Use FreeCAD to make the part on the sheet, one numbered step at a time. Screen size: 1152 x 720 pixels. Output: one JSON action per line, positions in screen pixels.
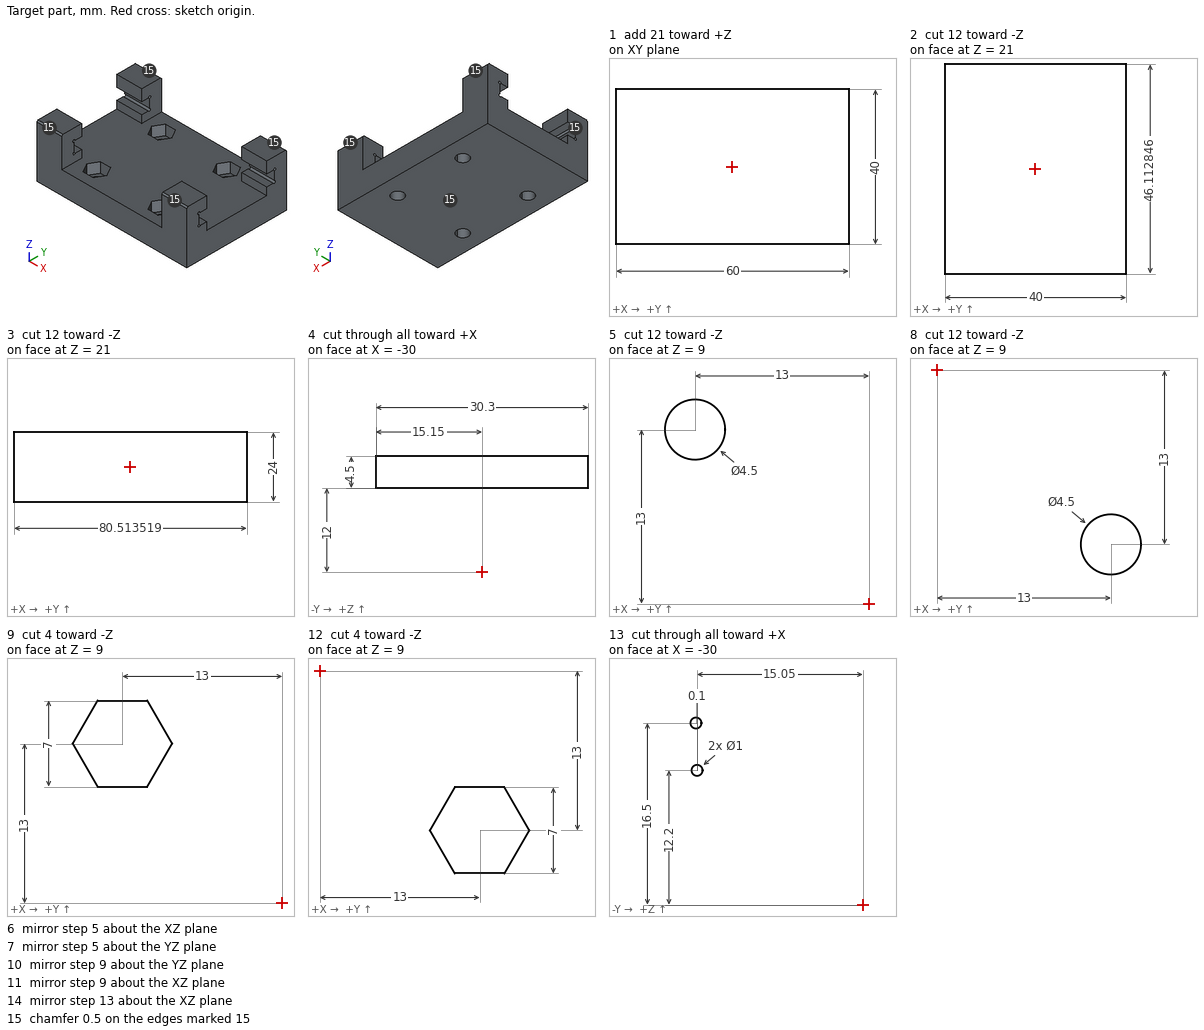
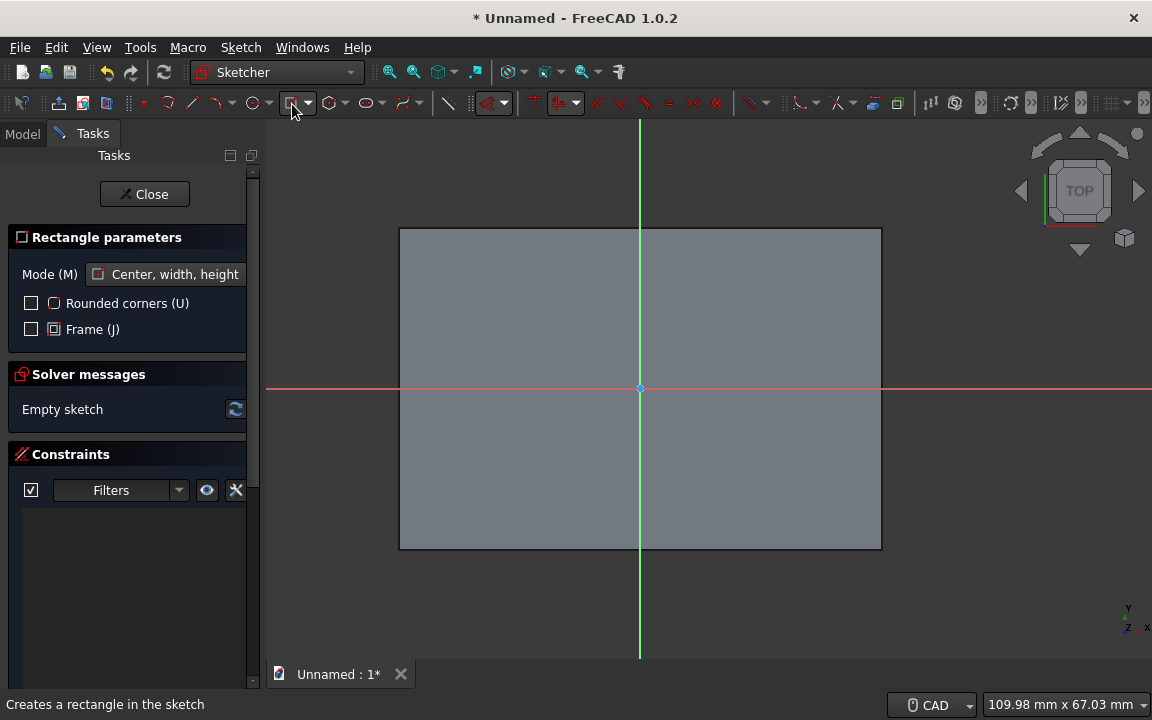
{"action": "left_click", "coordinate": [640, 389]}
{"action": "left_click", "coordinate": [801, 203]}
{"action": "key", "text": "Escape"}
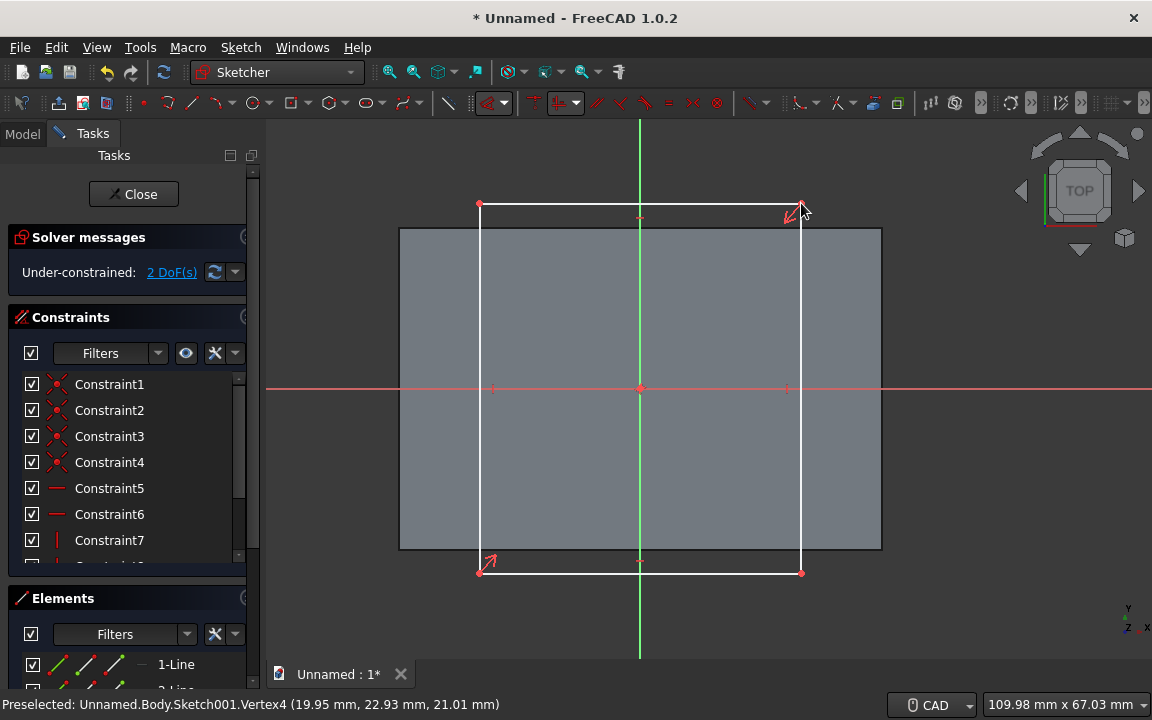
{"action": "left_click", "coordinate": [576, 574]}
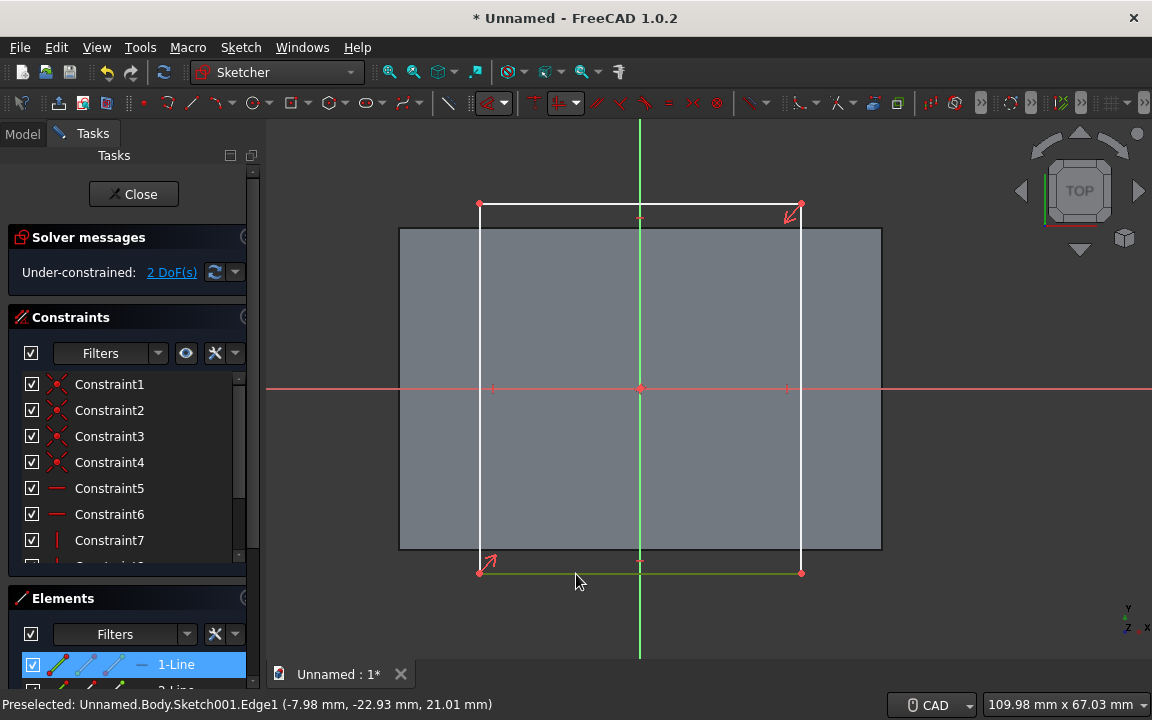
{"action": "key", "text": "l"}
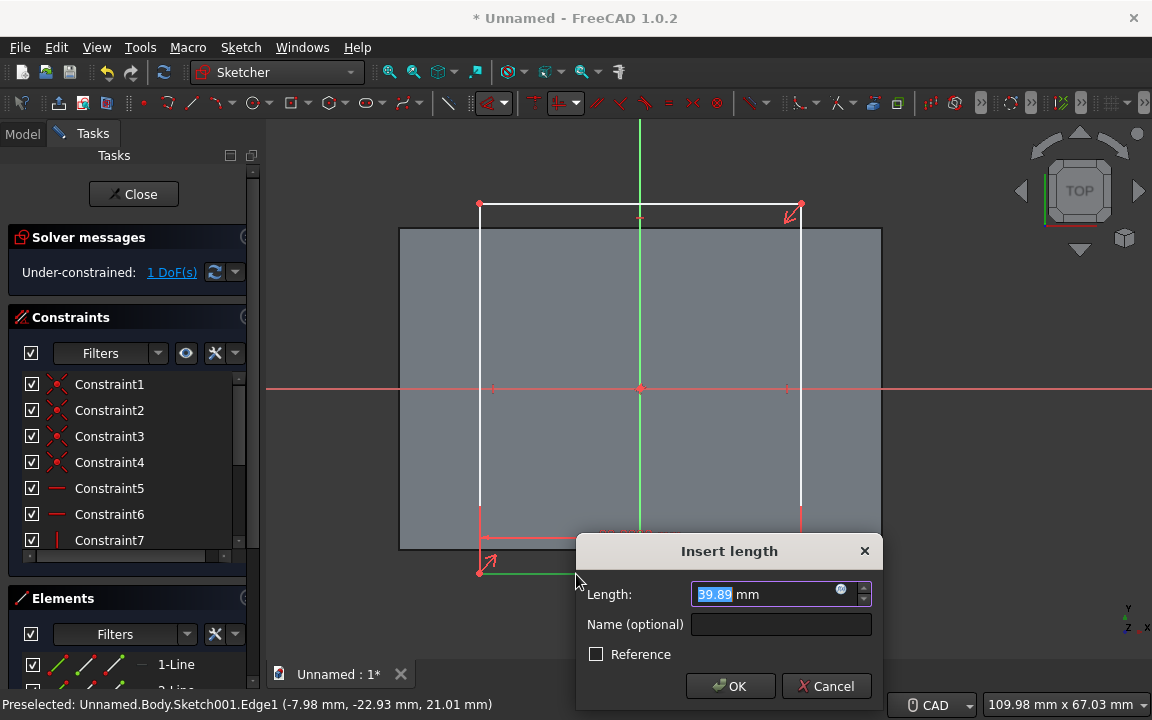
{"action": "type", "text": "40"}
{"action": "key", "text": "Return"}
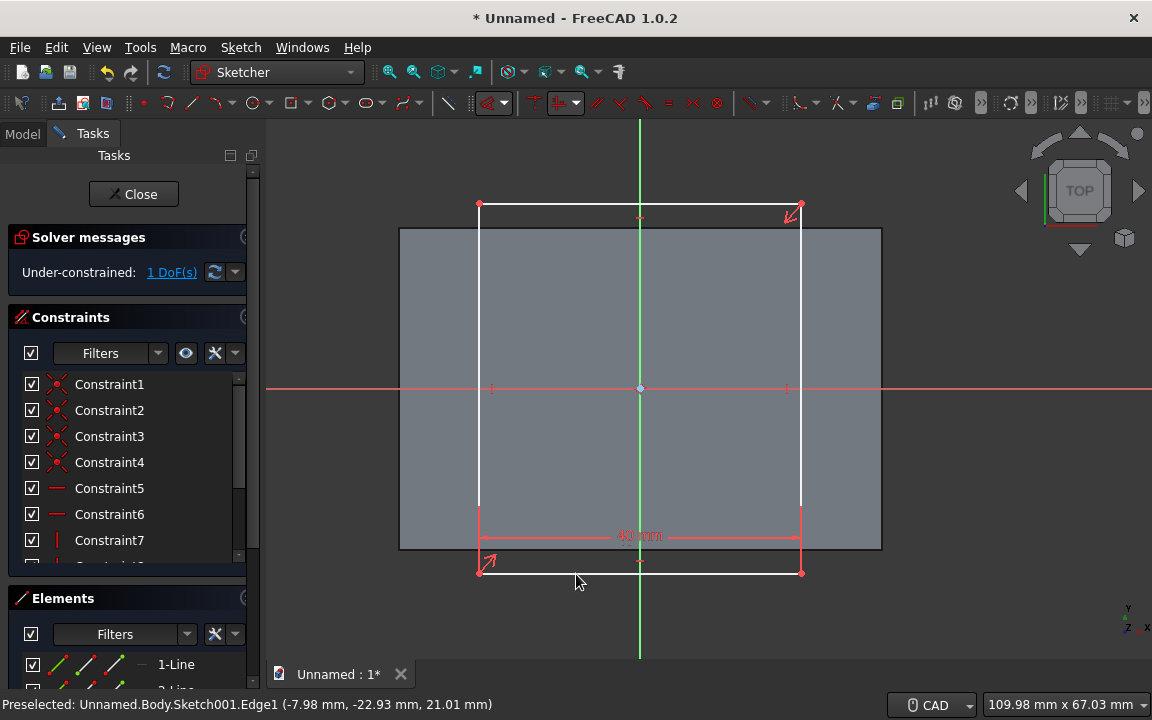
{"action": "left_click", "coordinate": [801, 463]}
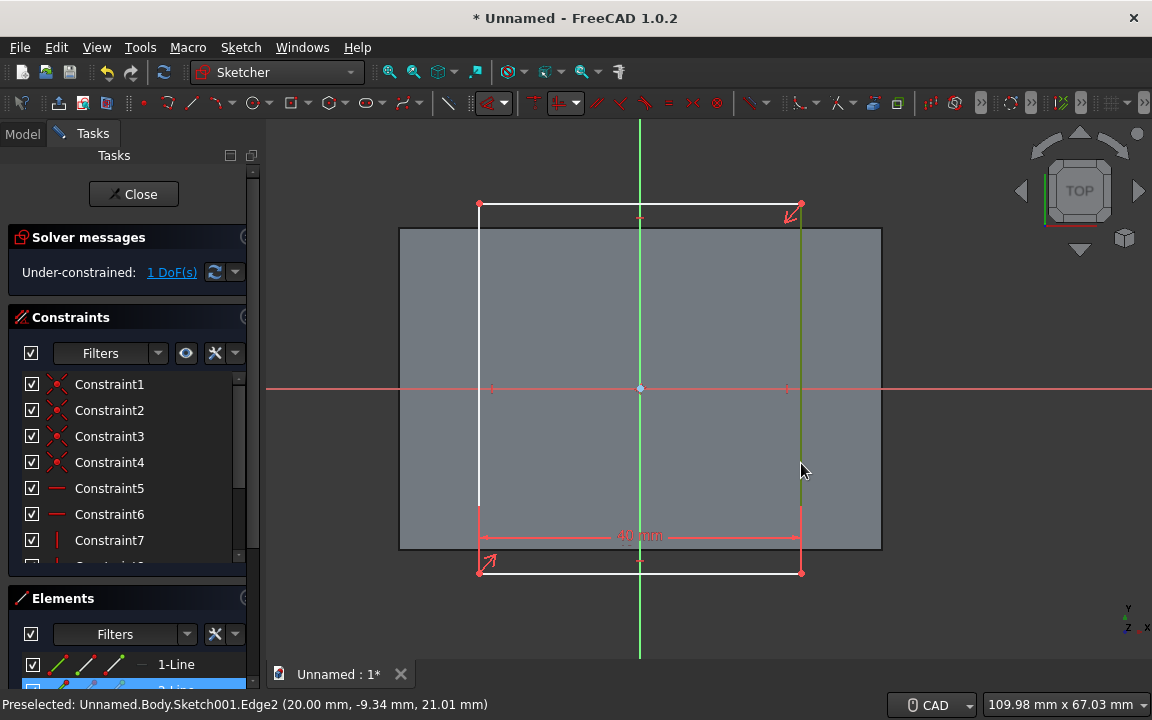
{"action": "left_click", "coordinate": [506, 104]}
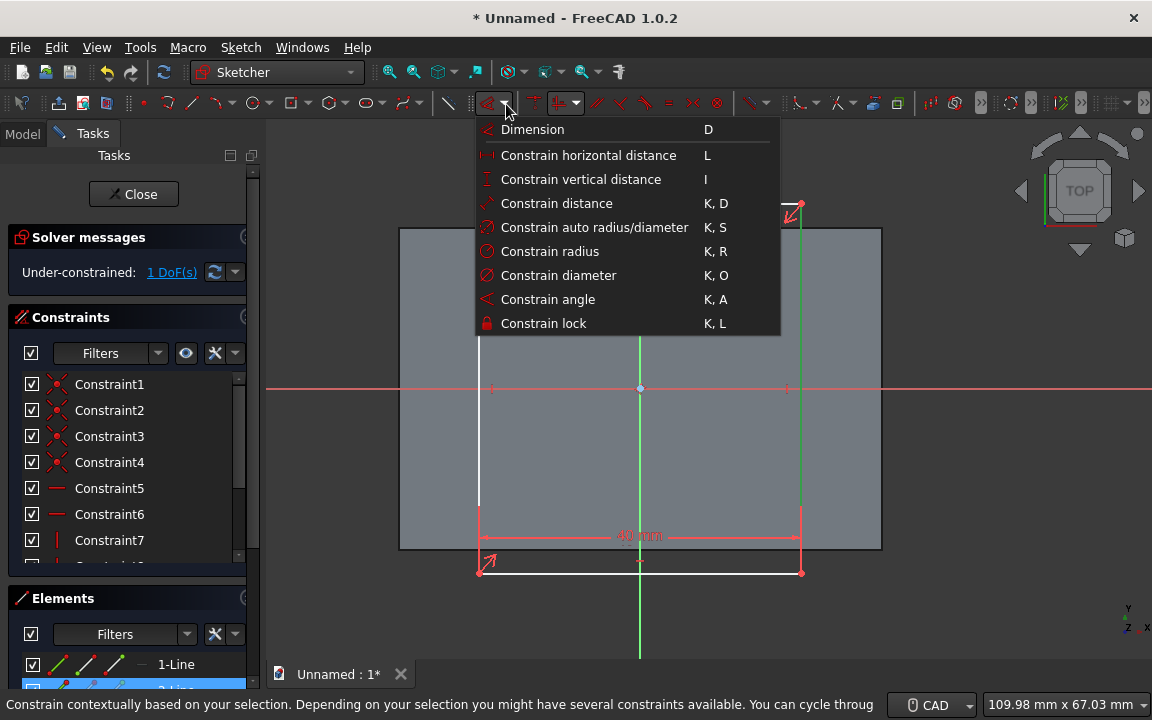
{"action": "left_click", "coordinate": [628, 179]}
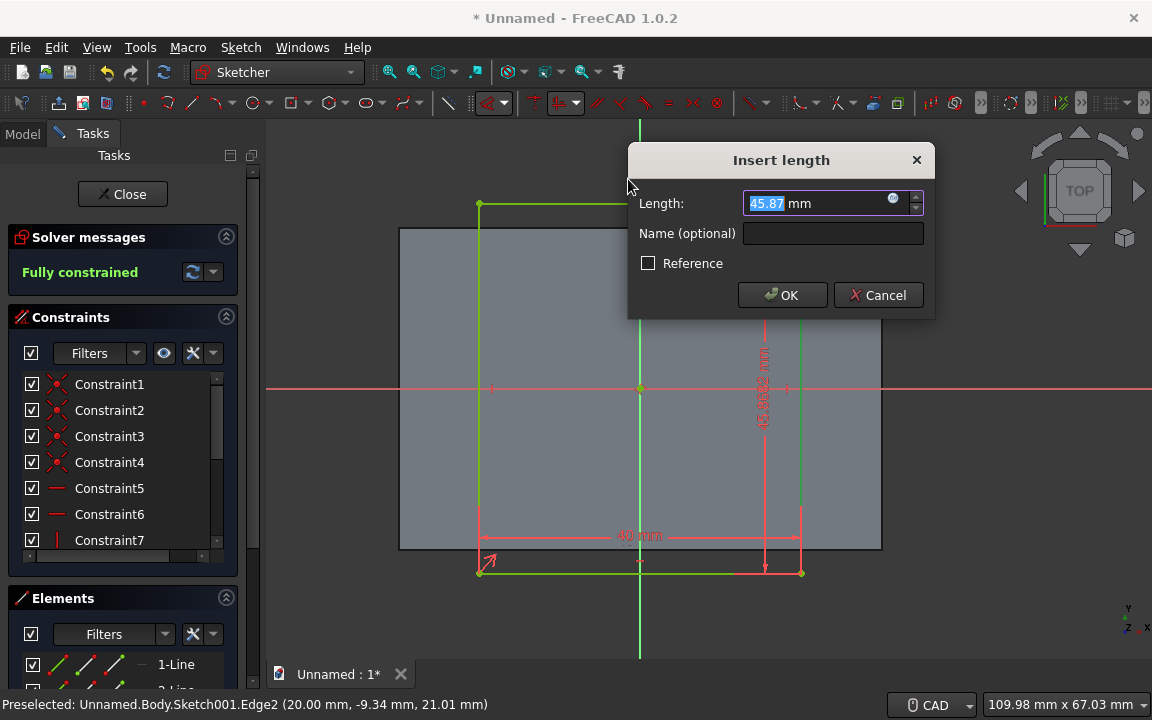
{"action": "type", "text": "46.112846"}
{"action": "key", "text": "Return"}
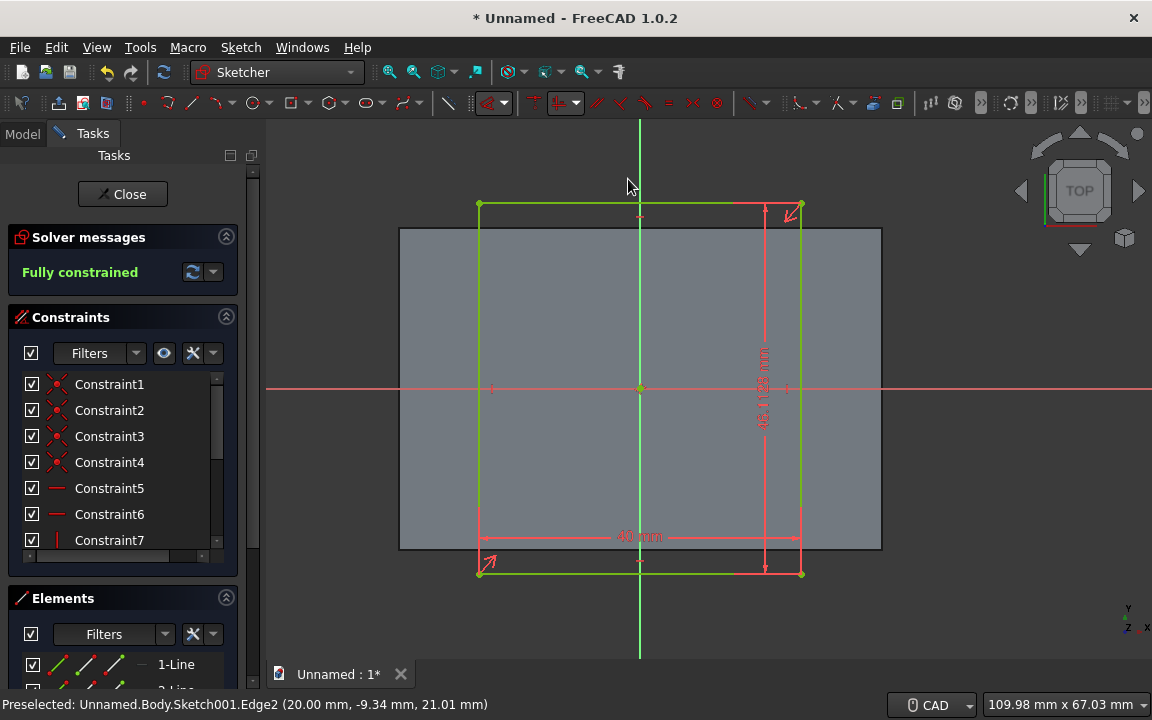
{"action": "left_click", "coordinate": [123, 194]}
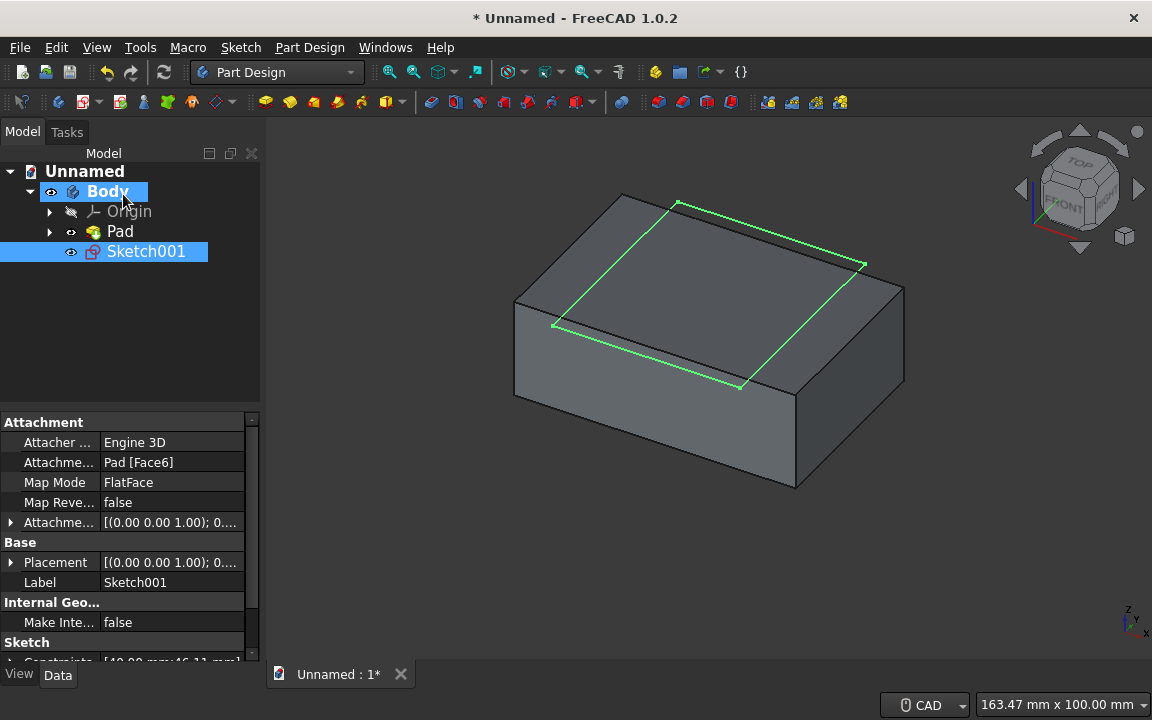
{"action": "left_click", "coordinate": [432, 102]}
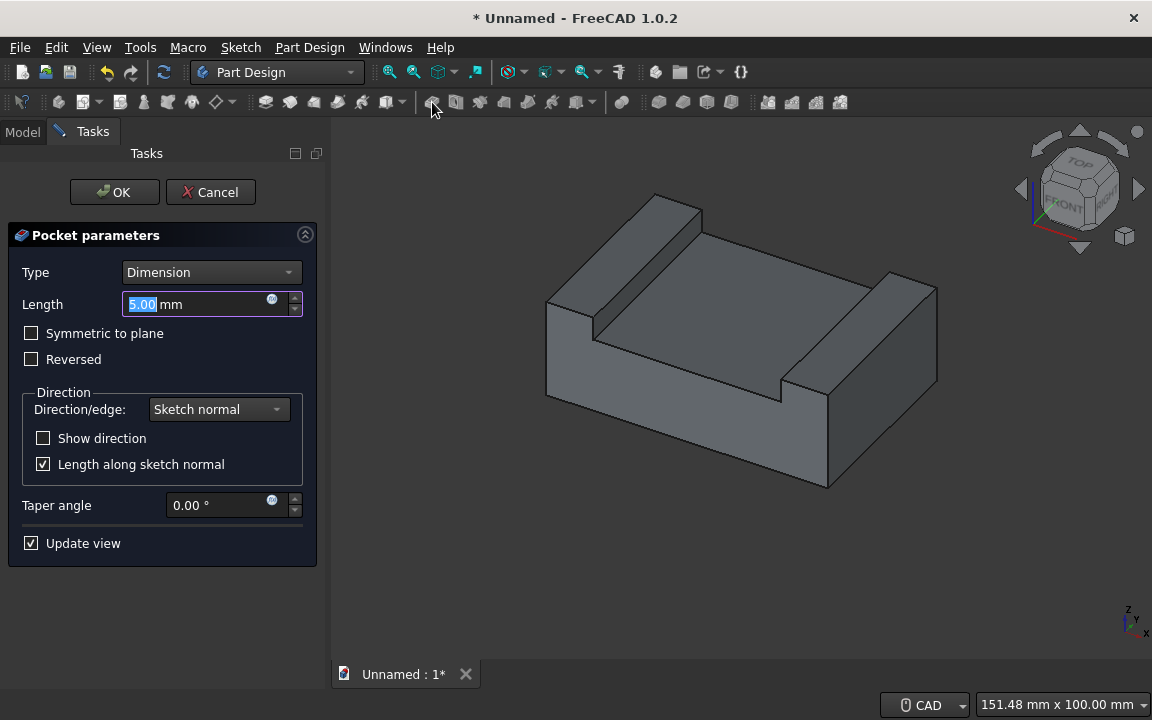
{"action": "type", "text": "12"}
{"action": "key", "text": "Tab"}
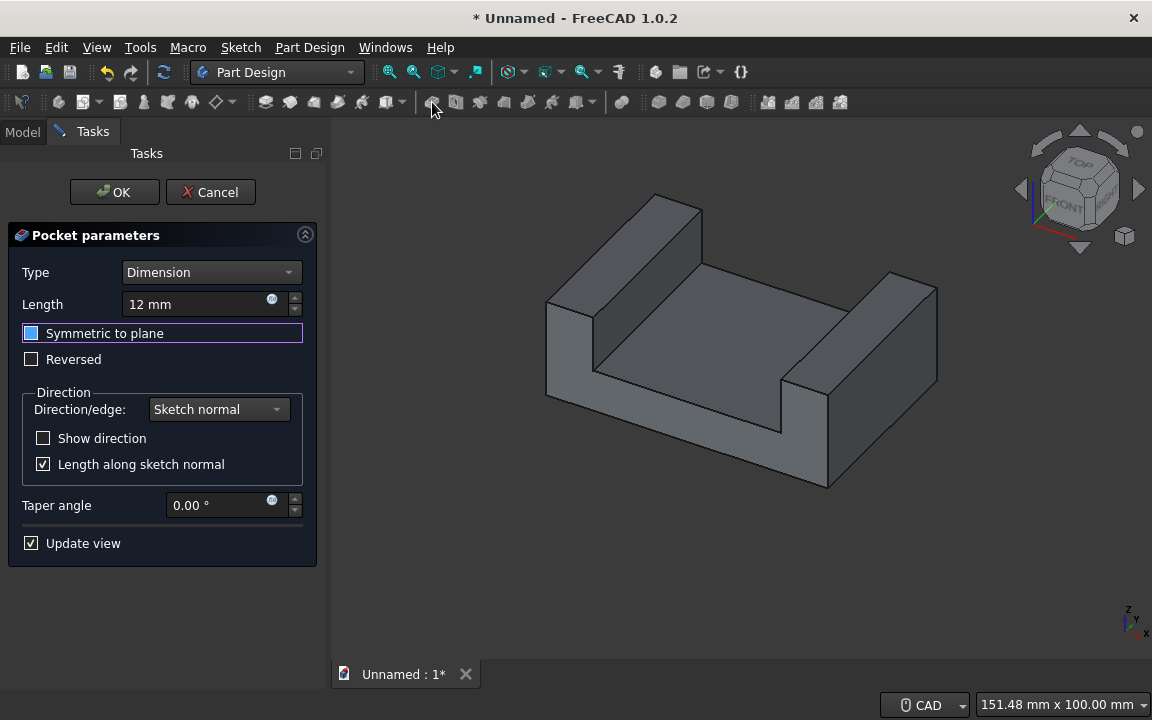
{"action": "left_click", "coordinate": [115, 192]}